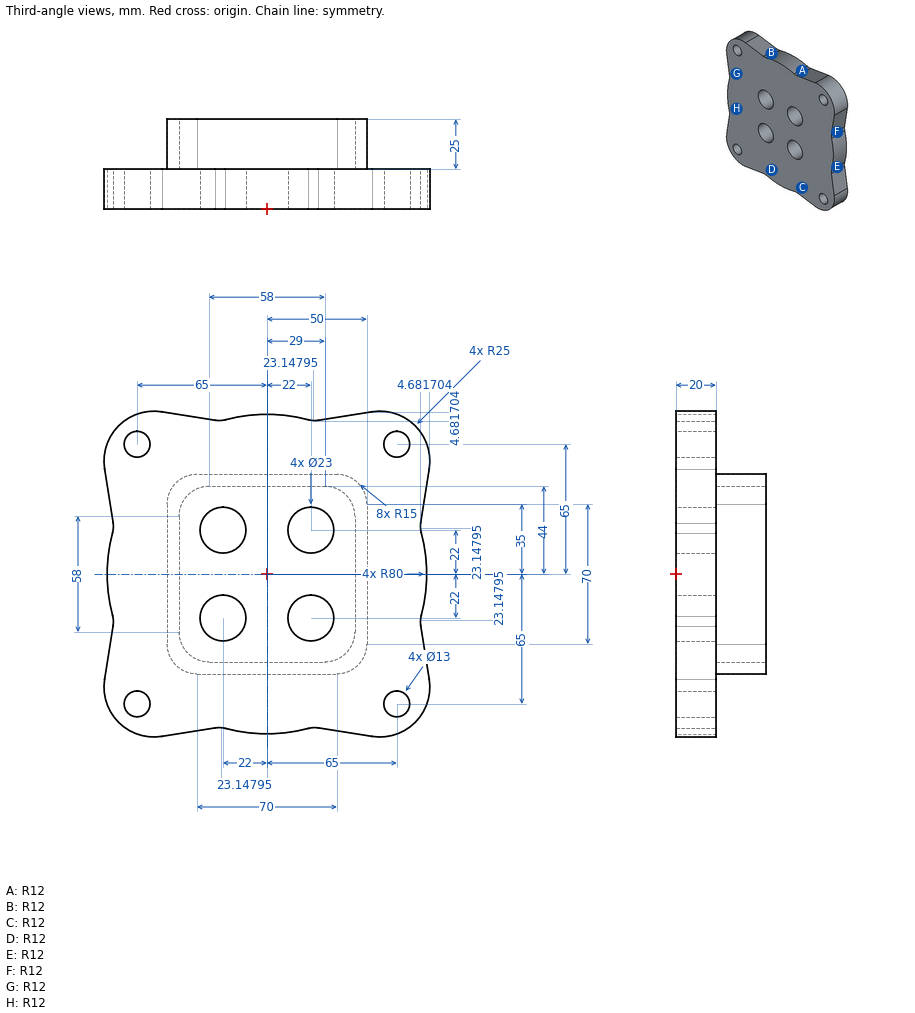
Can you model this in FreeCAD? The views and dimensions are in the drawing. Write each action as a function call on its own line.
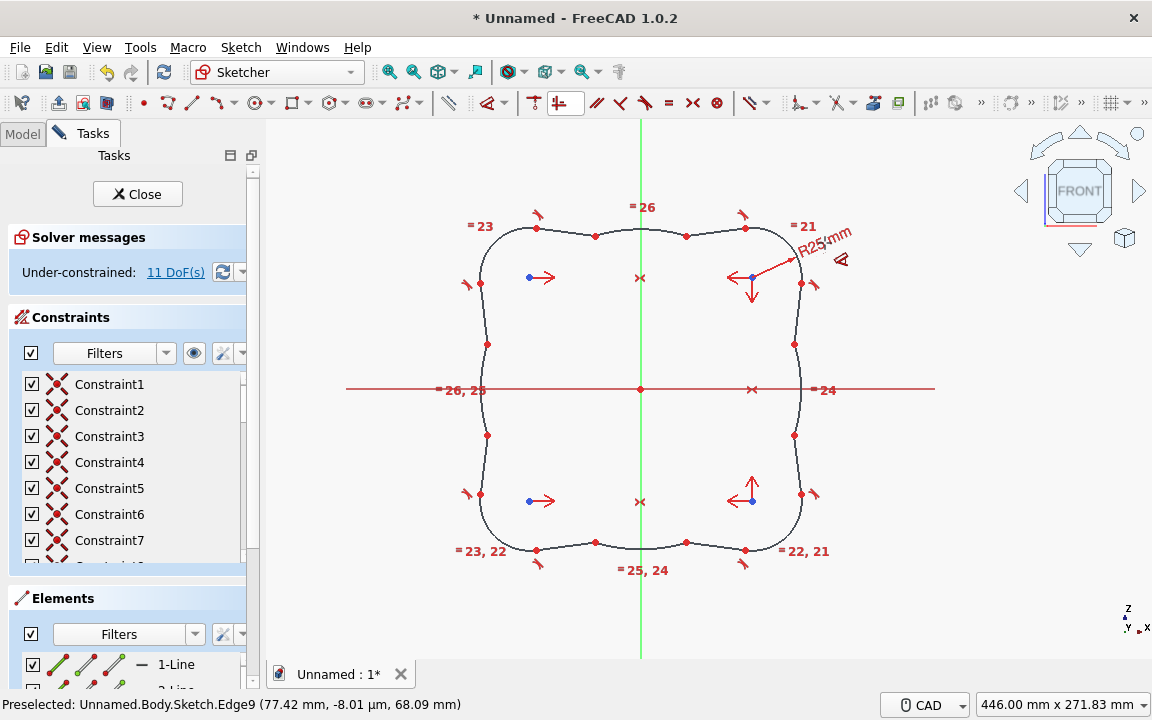
click(800, 409)
click(832, 413)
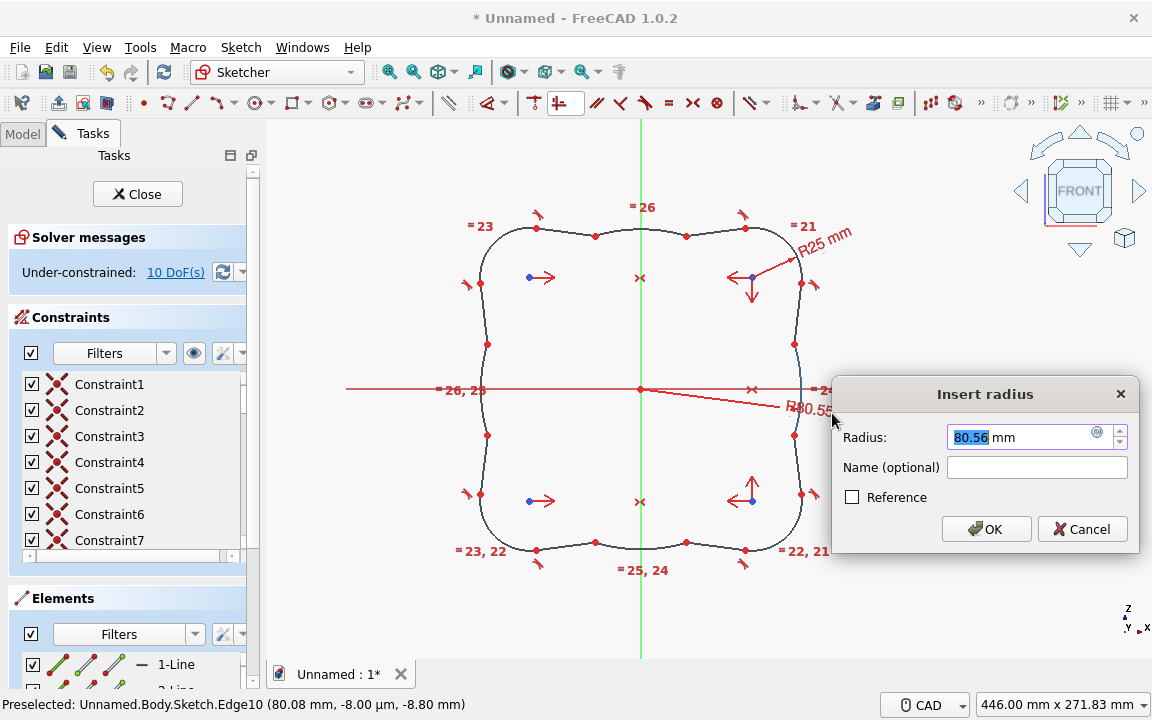
text(80)
key(Return)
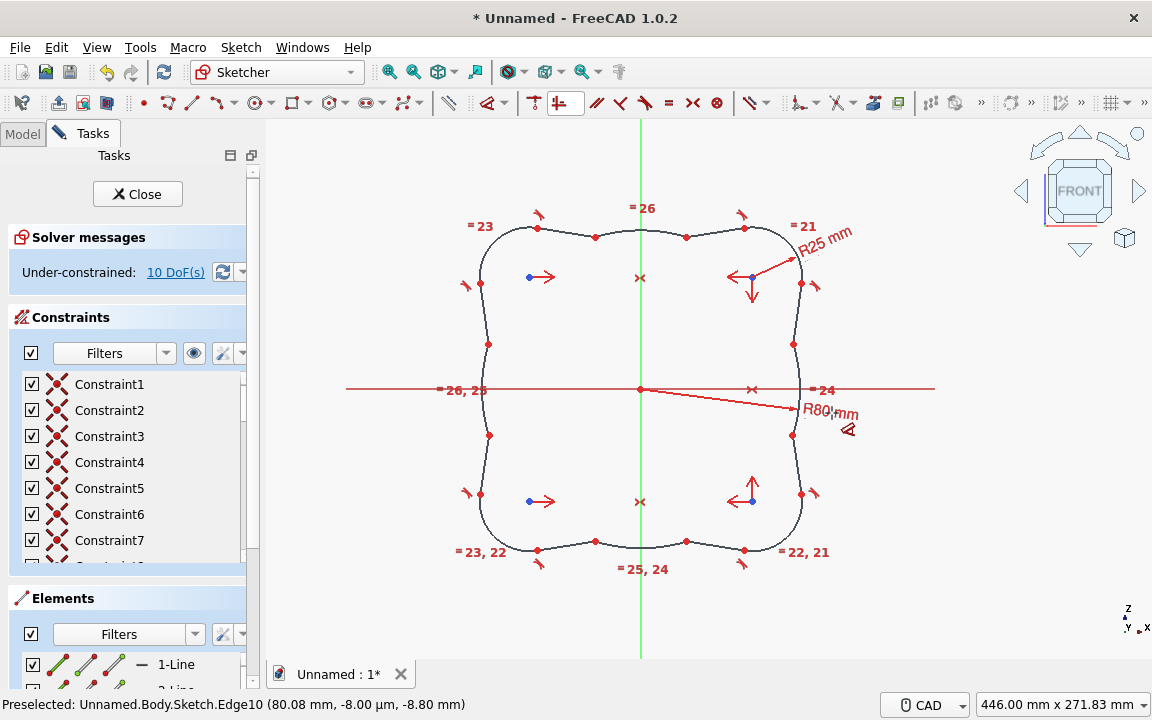
click(687, 237)
click(664, 203)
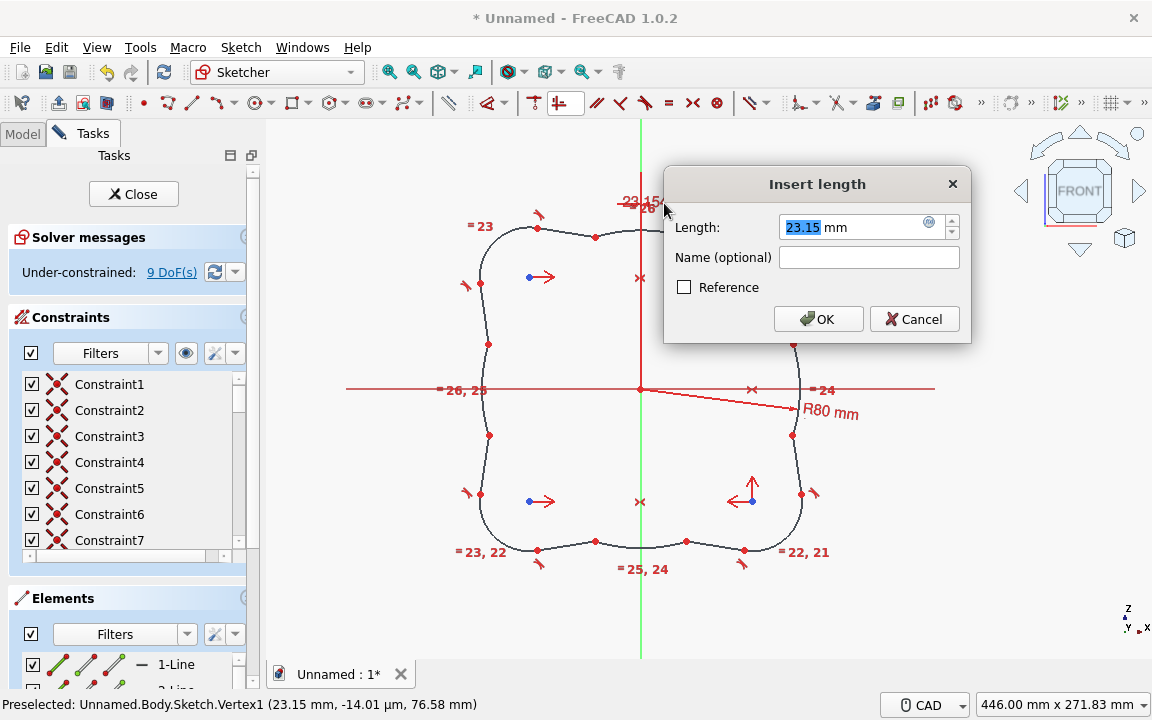
text(23.14795)
key(Return)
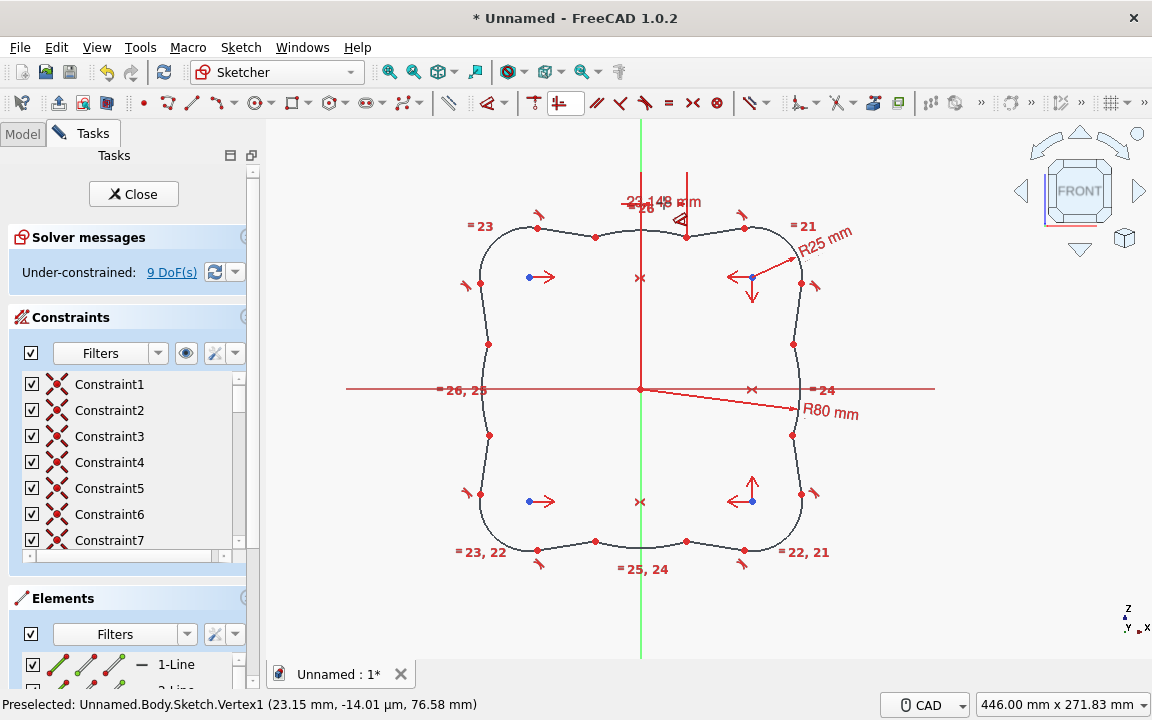
click(793, 344)
click(827, 367)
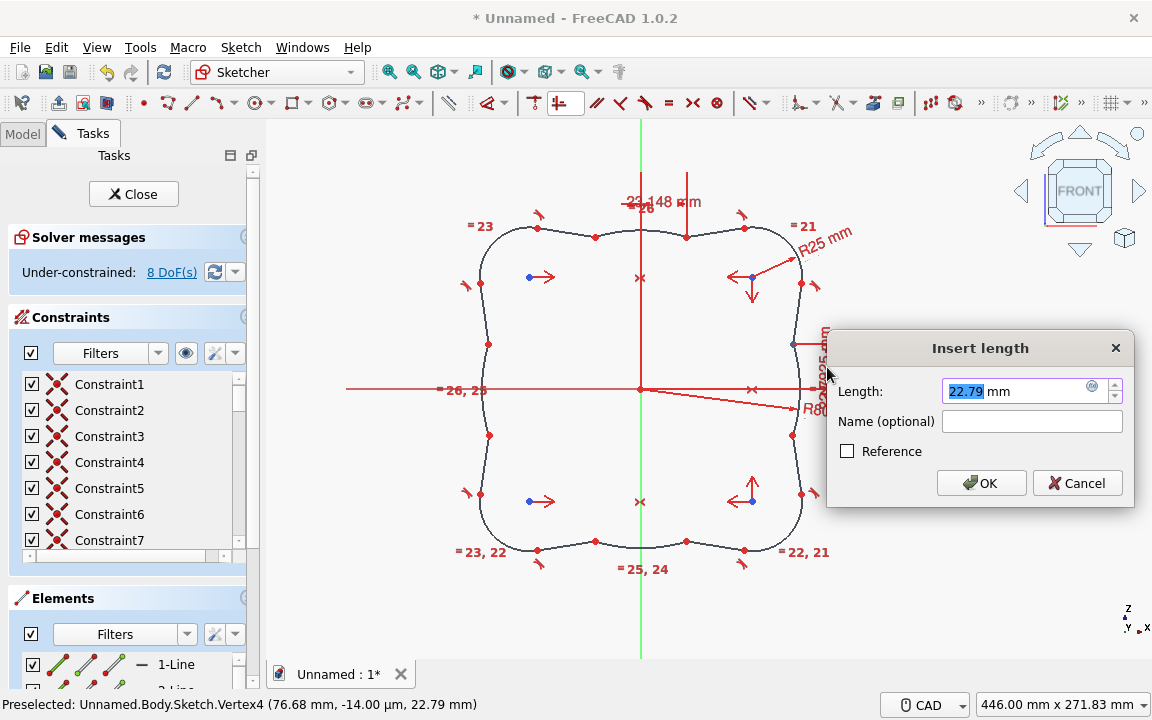
text(23.14795)
key(Return)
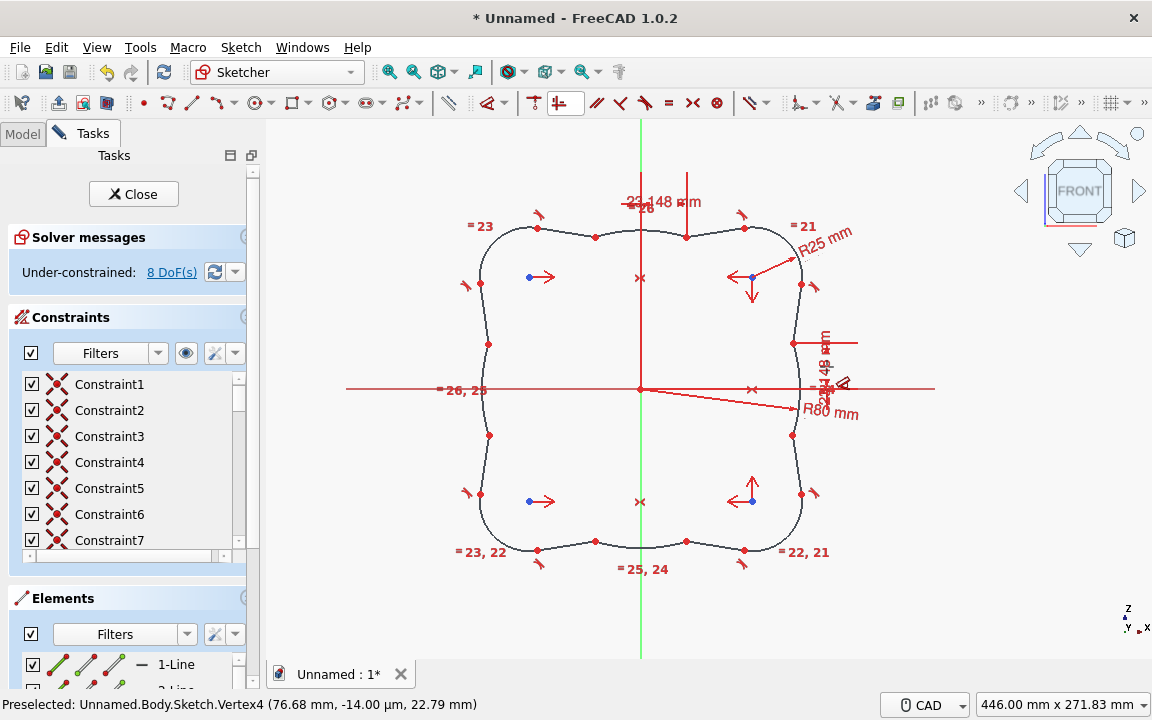
click(793, 436)
click(607, 413)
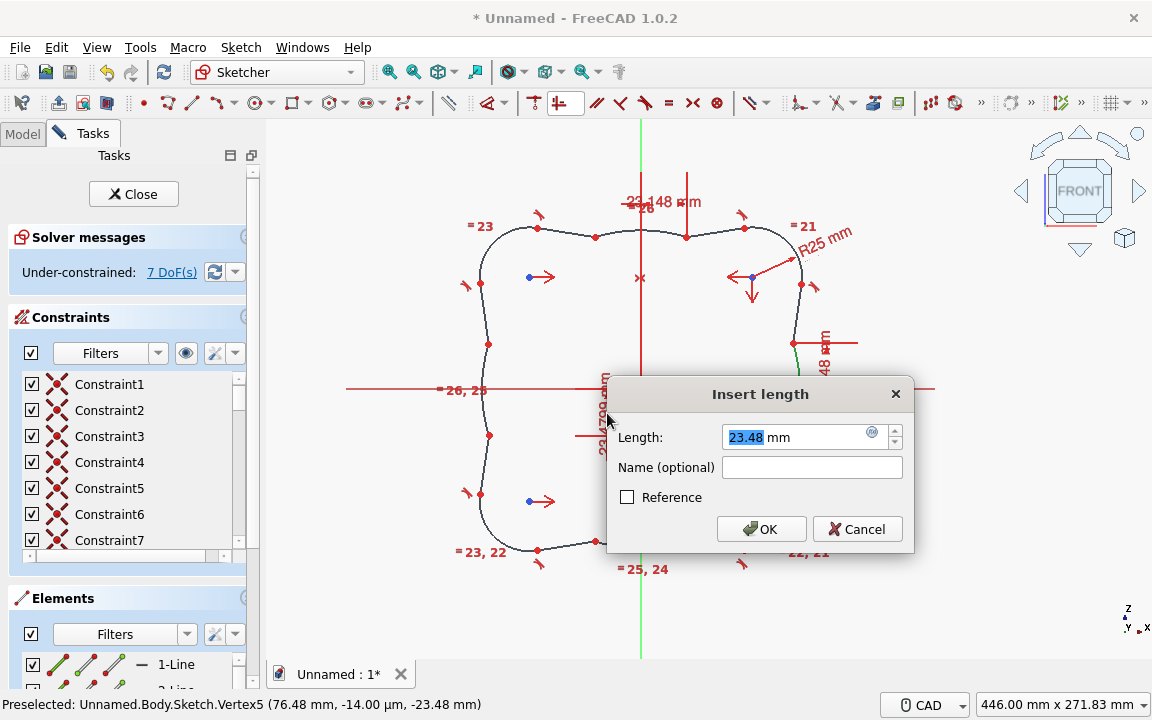
text(23.14795)
key(Return)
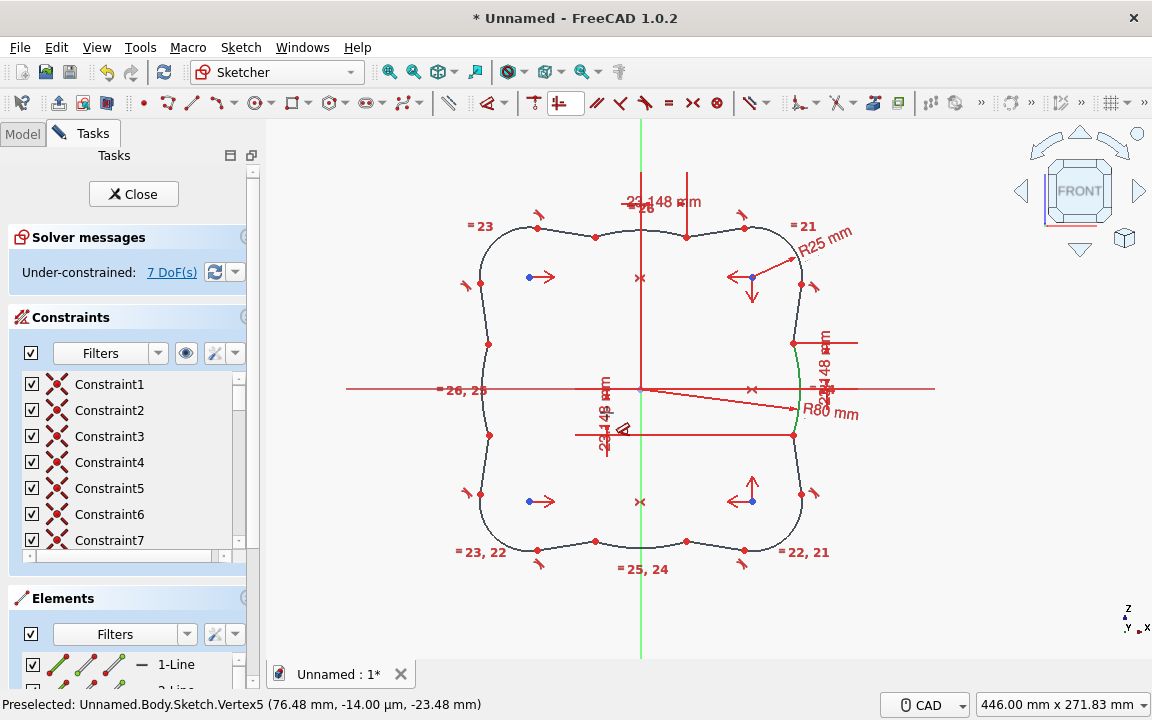
click(687, 541)
click(664, 575)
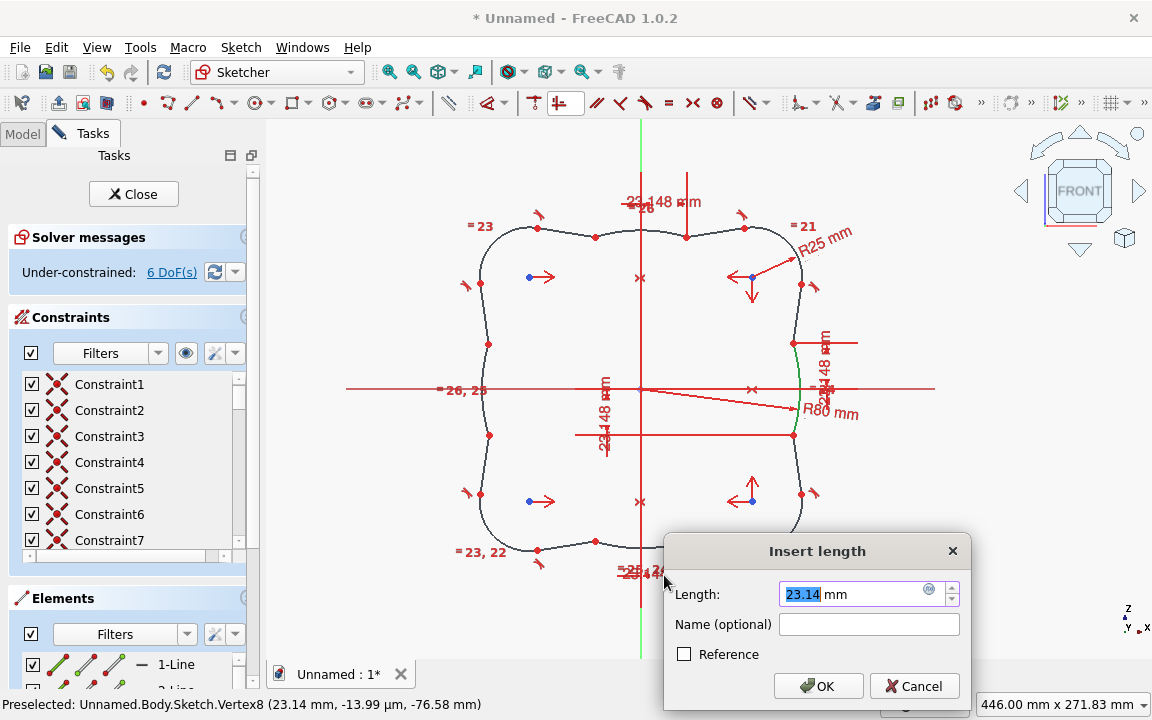
text(23.14795)
key(Return)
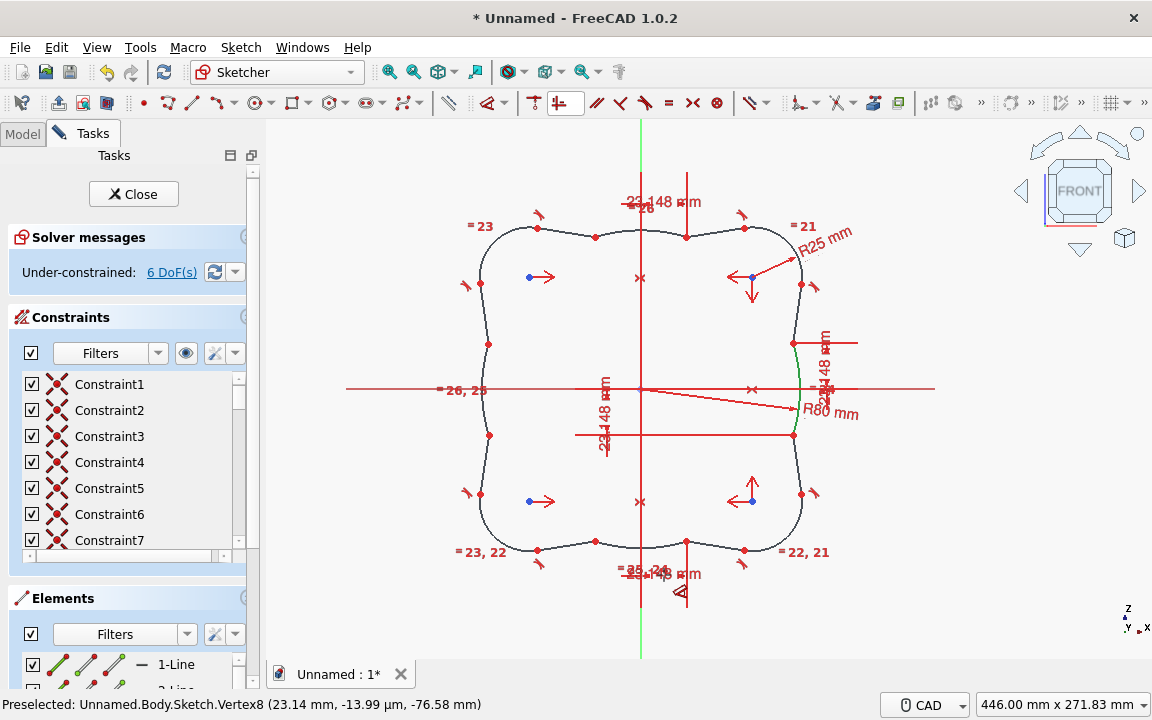
click(595, 541)
click(618, 355)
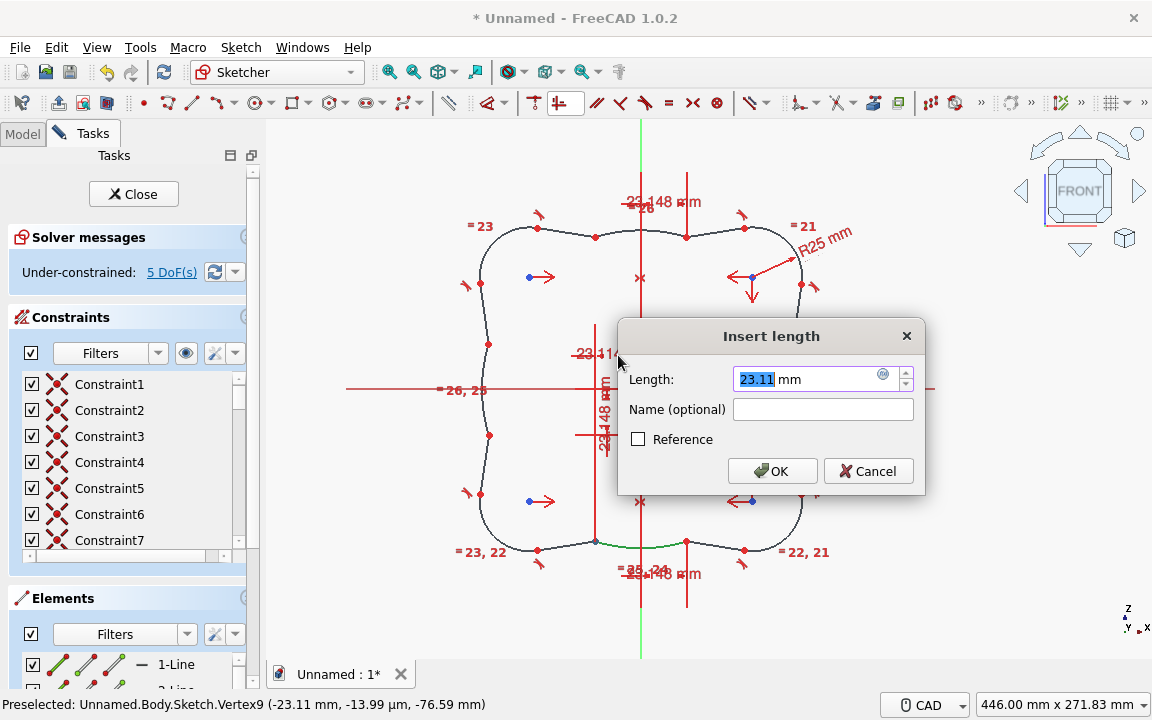
text(23.14795)
key(Return)